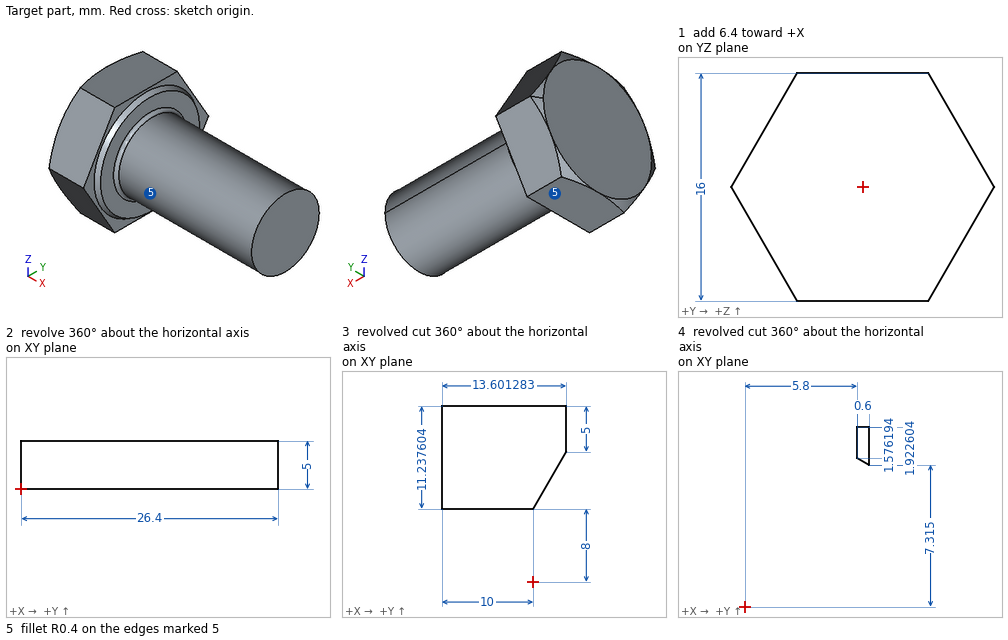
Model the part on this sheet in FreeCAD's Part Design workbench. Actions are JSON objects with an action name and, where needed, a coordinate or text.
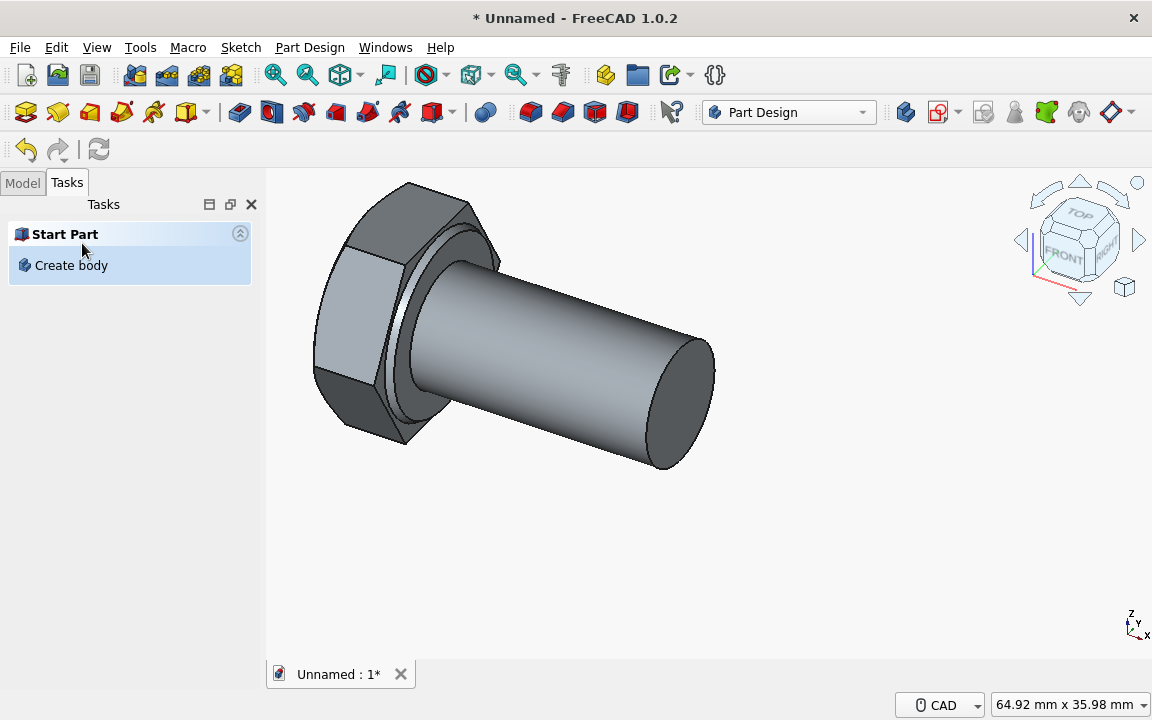
{"action": "left_click", "coordinate": [276, 76]}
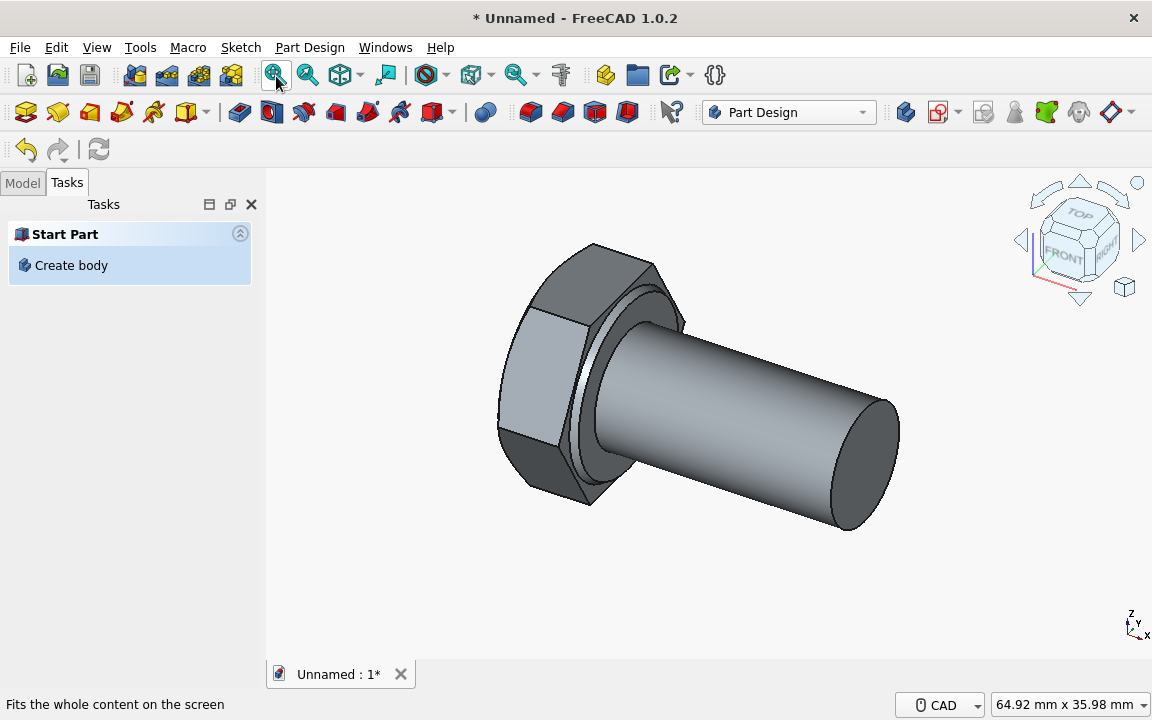
{"action": "key", "text": "0"}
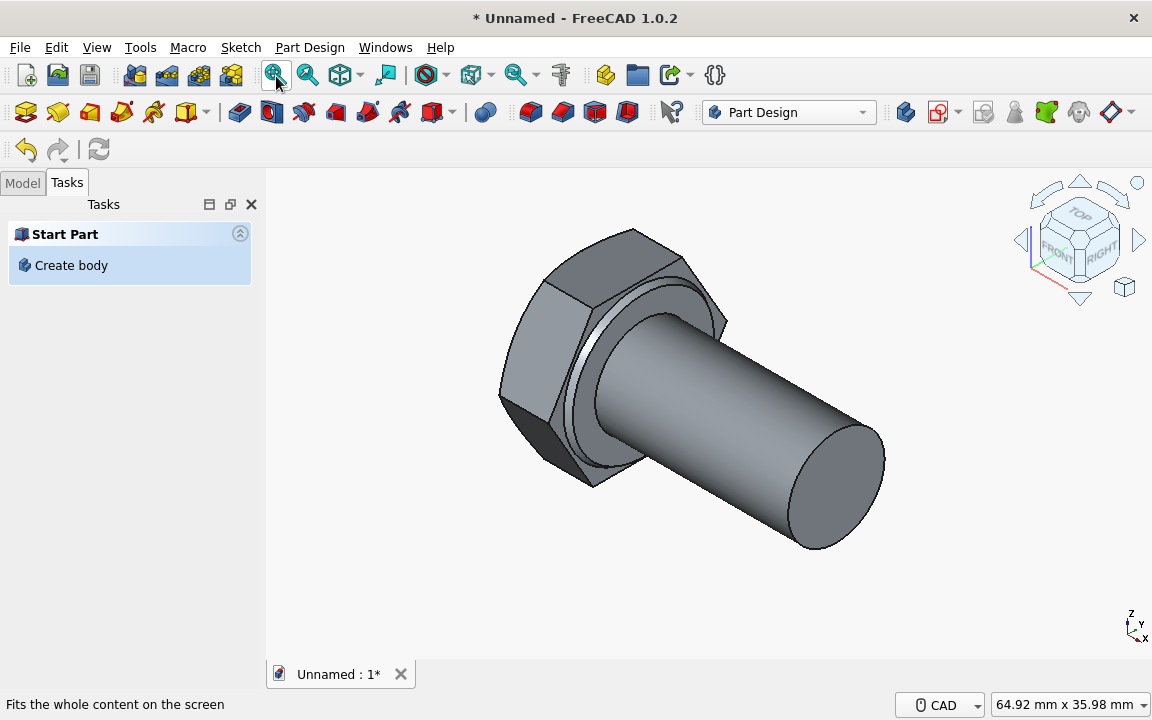
{"action": "key", "text": "2"}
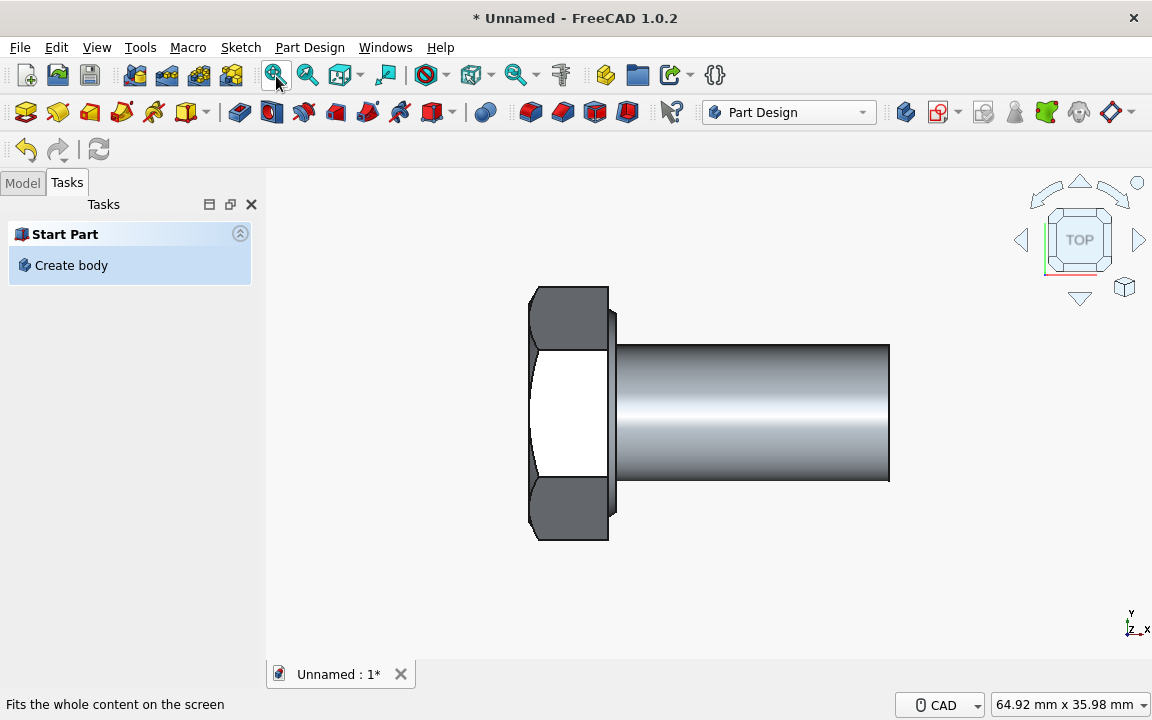
{"action": "key", "text": "1"}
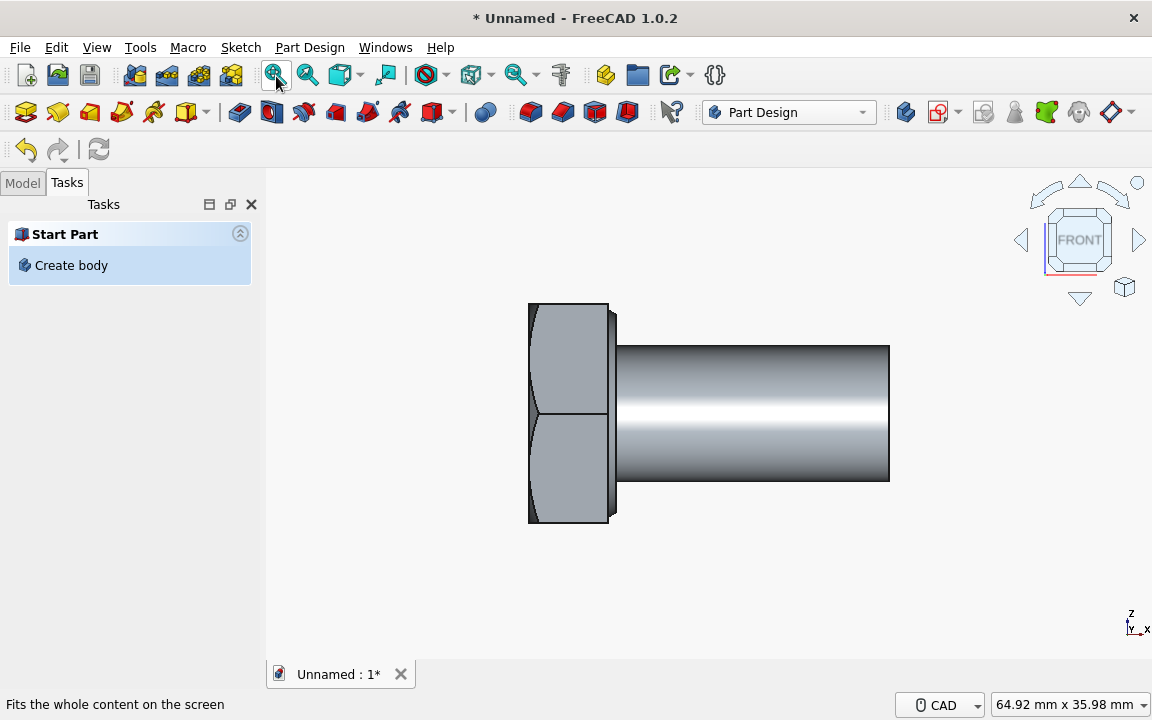
{"action": "left_click", "coordinate": [276, 76]}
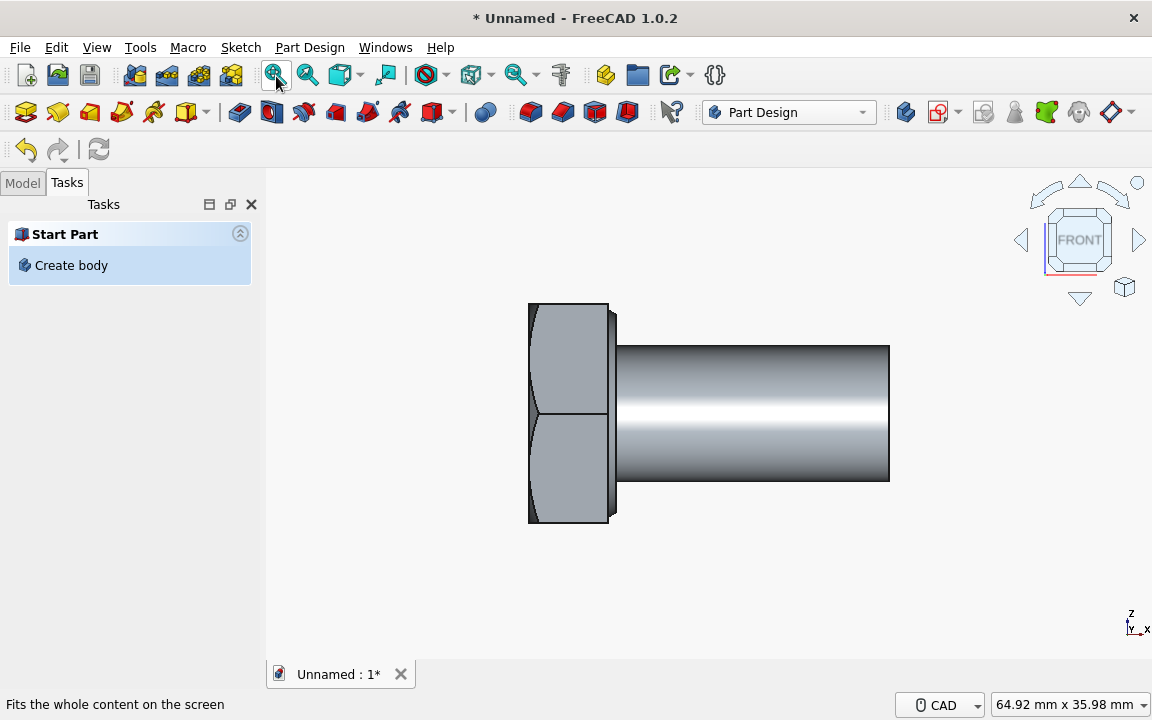
{"action": "key", "text": "3"}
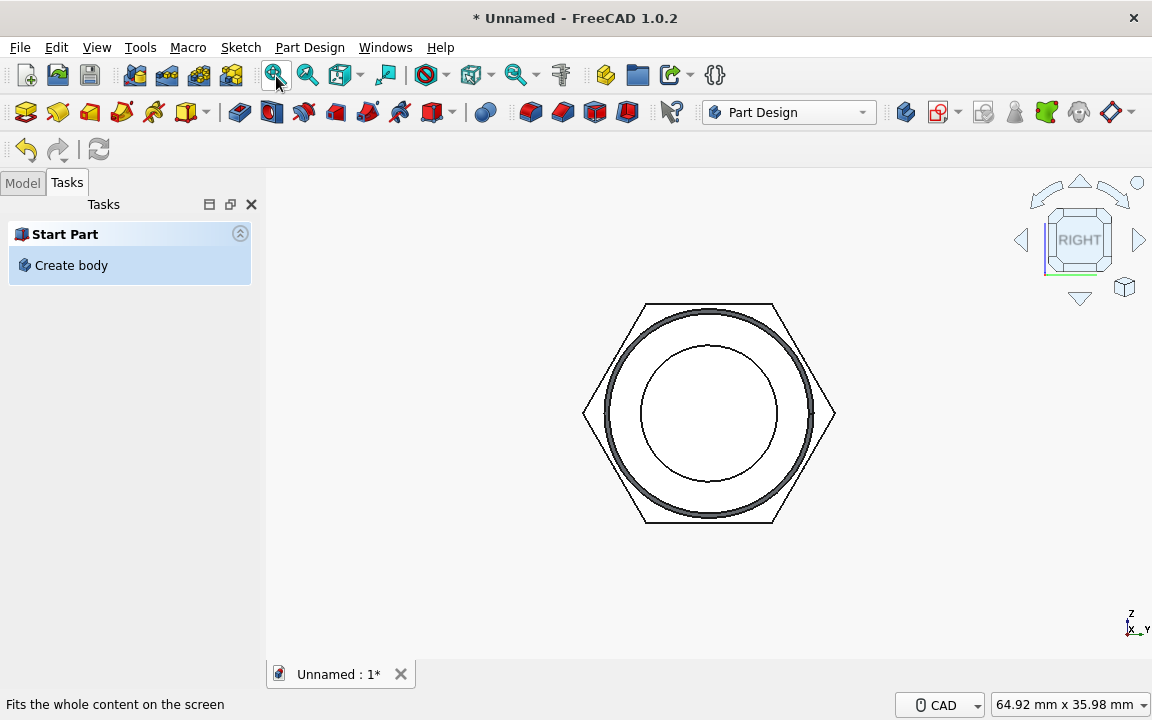
{"action": "left_click", "coordinate": [276, 76]}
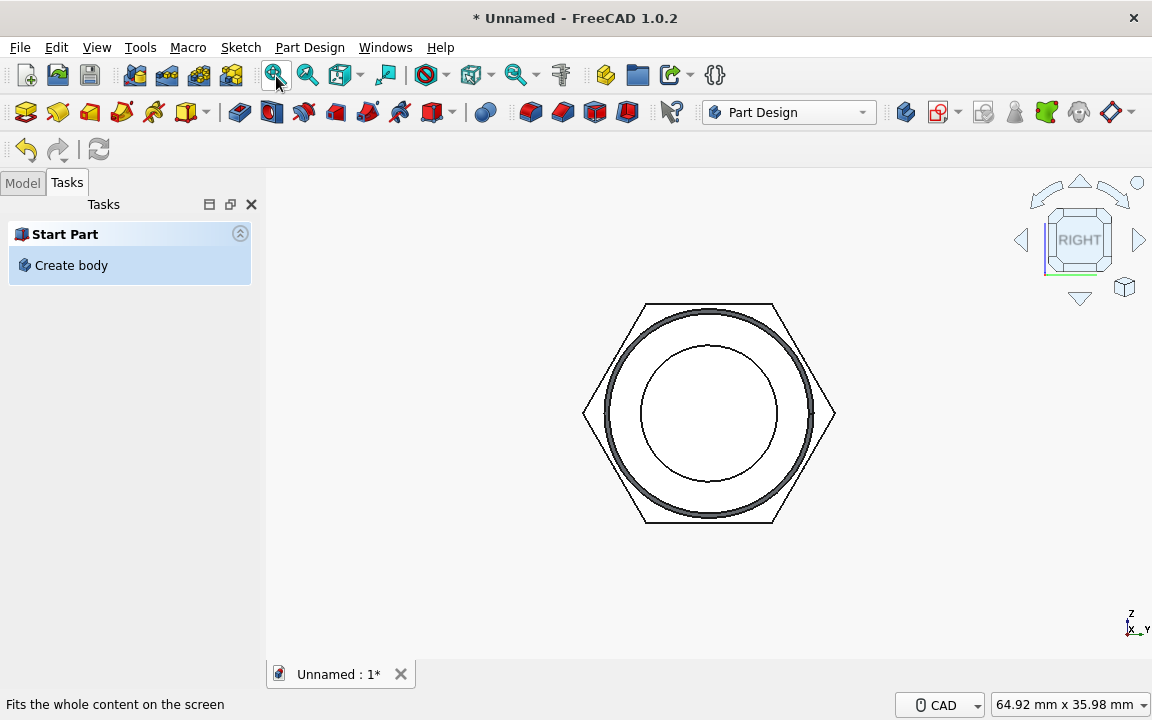
{"action": "key", "text": "5"}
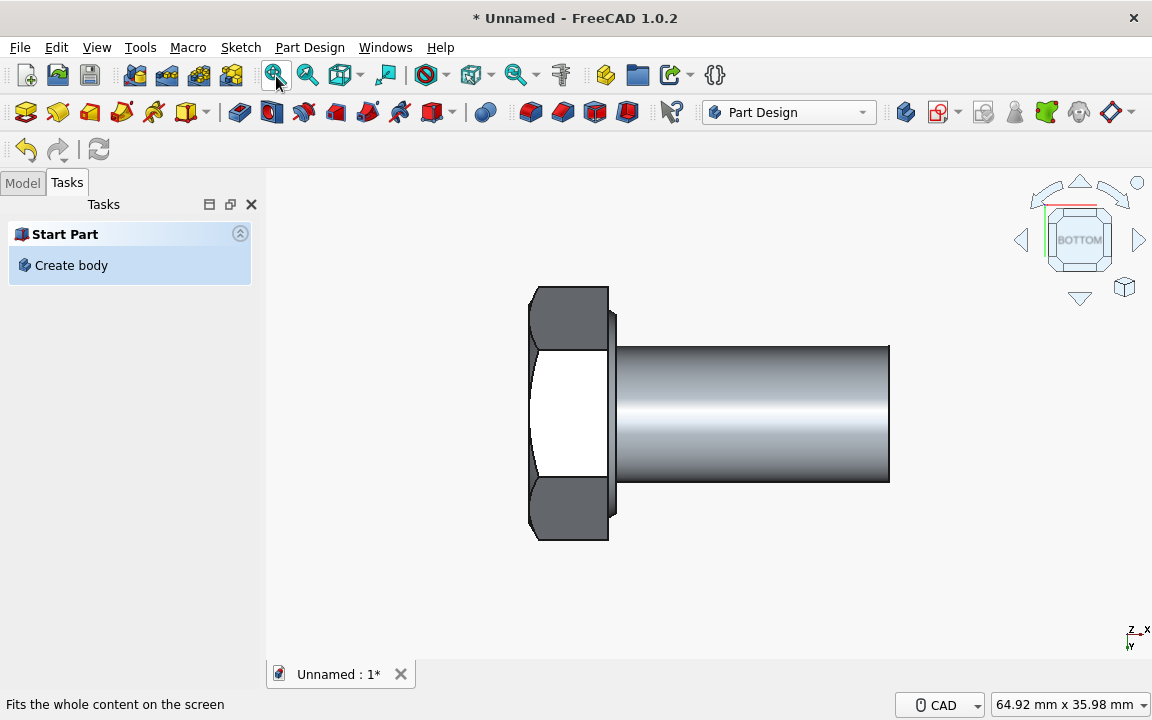
{"action": "key", "text": "4"}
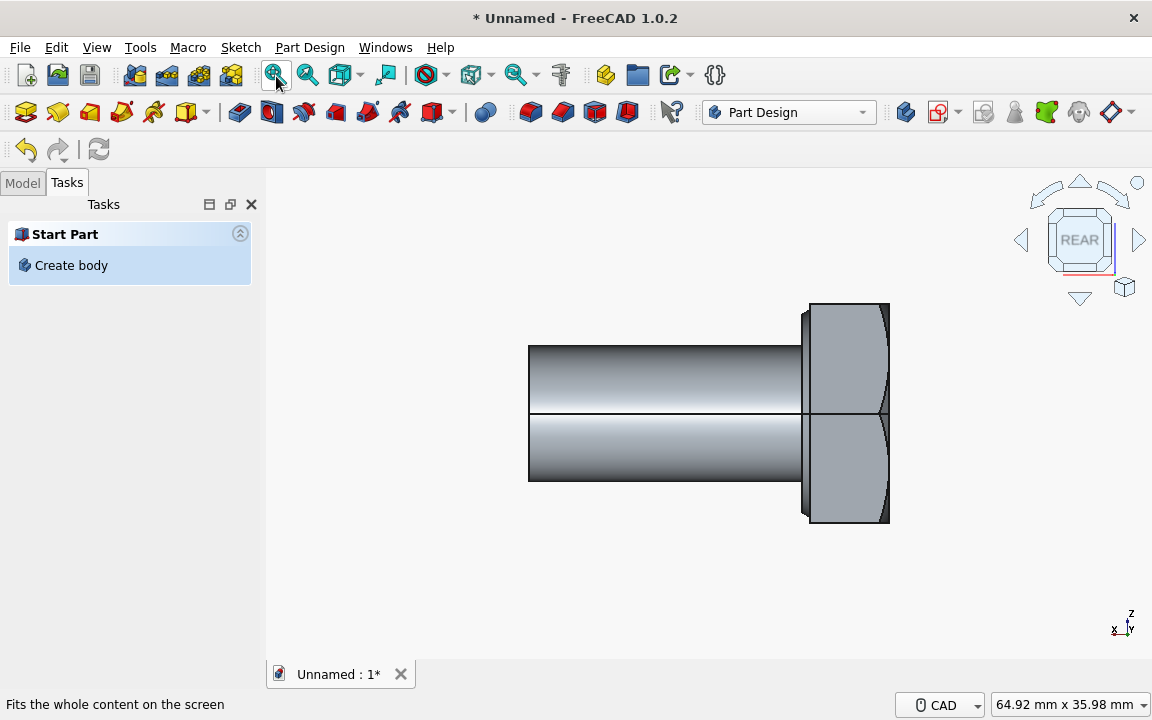
{"action": "left_click", "coordinate": [276, 76]}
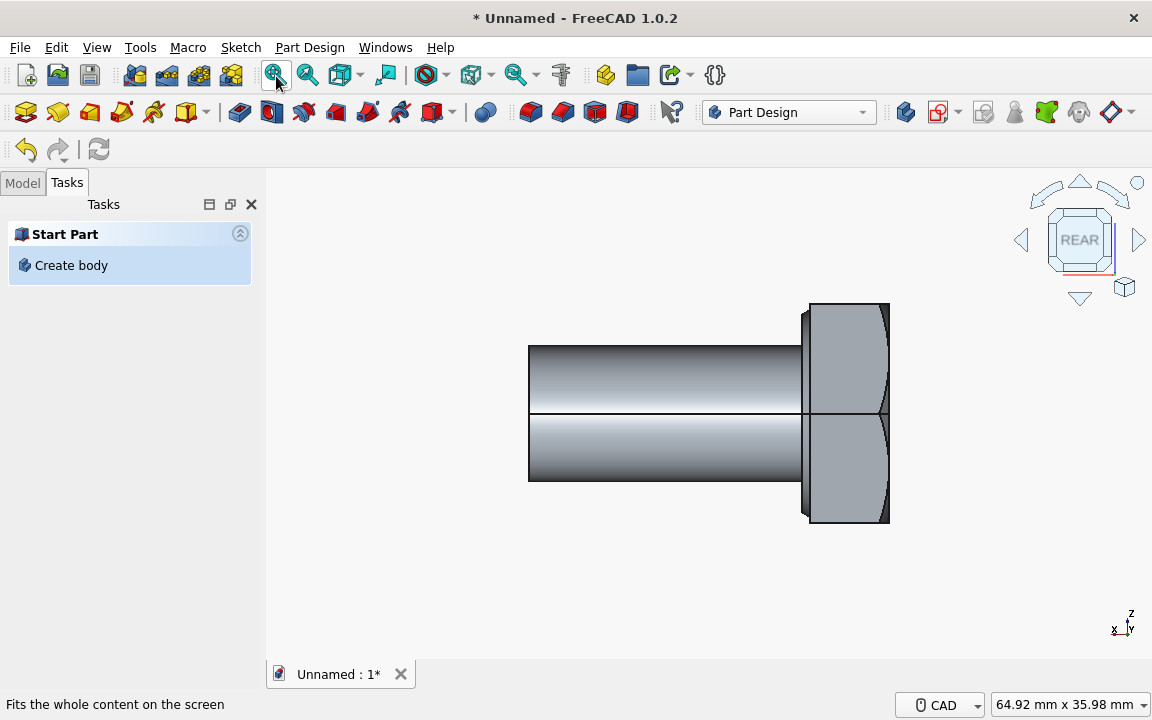
{"action": "key", "text": "6"}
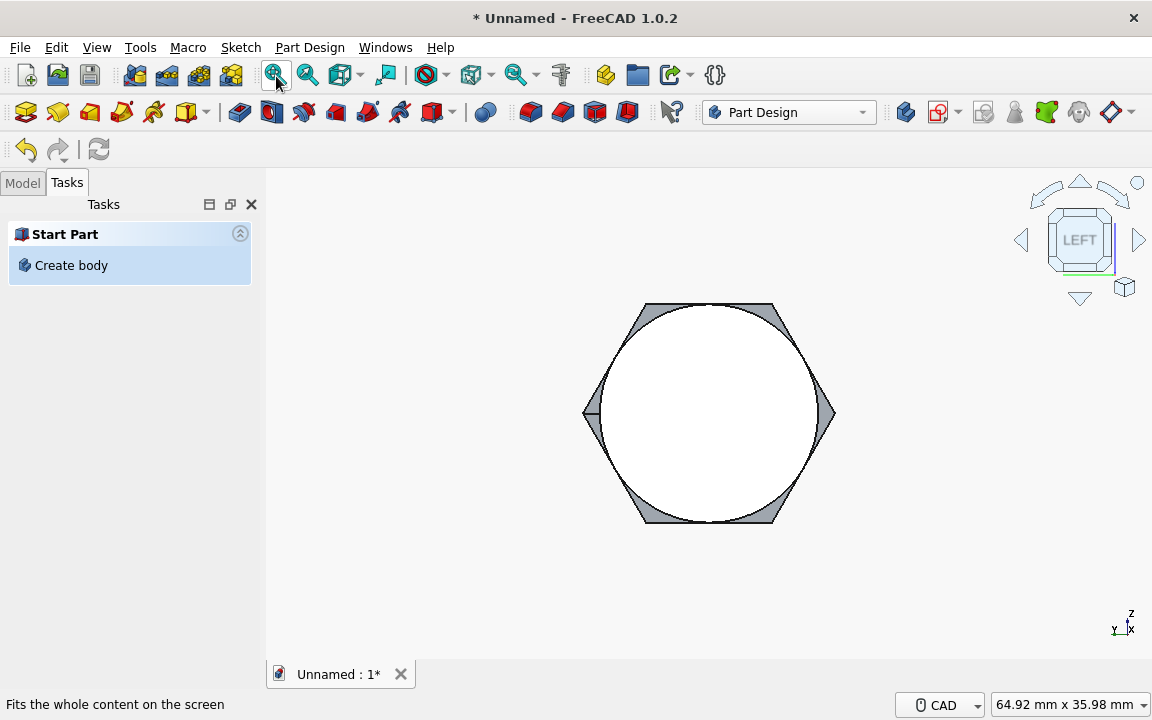
{"action": "left_click", "coordinate": [276, 76]}